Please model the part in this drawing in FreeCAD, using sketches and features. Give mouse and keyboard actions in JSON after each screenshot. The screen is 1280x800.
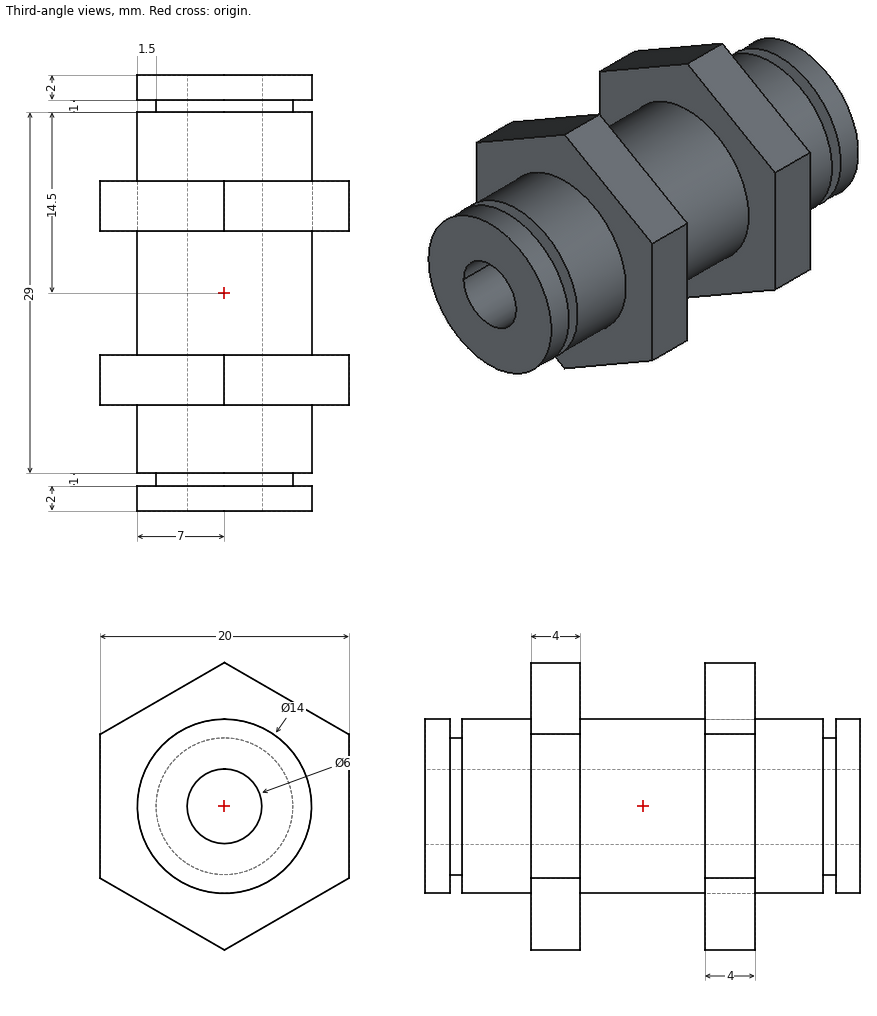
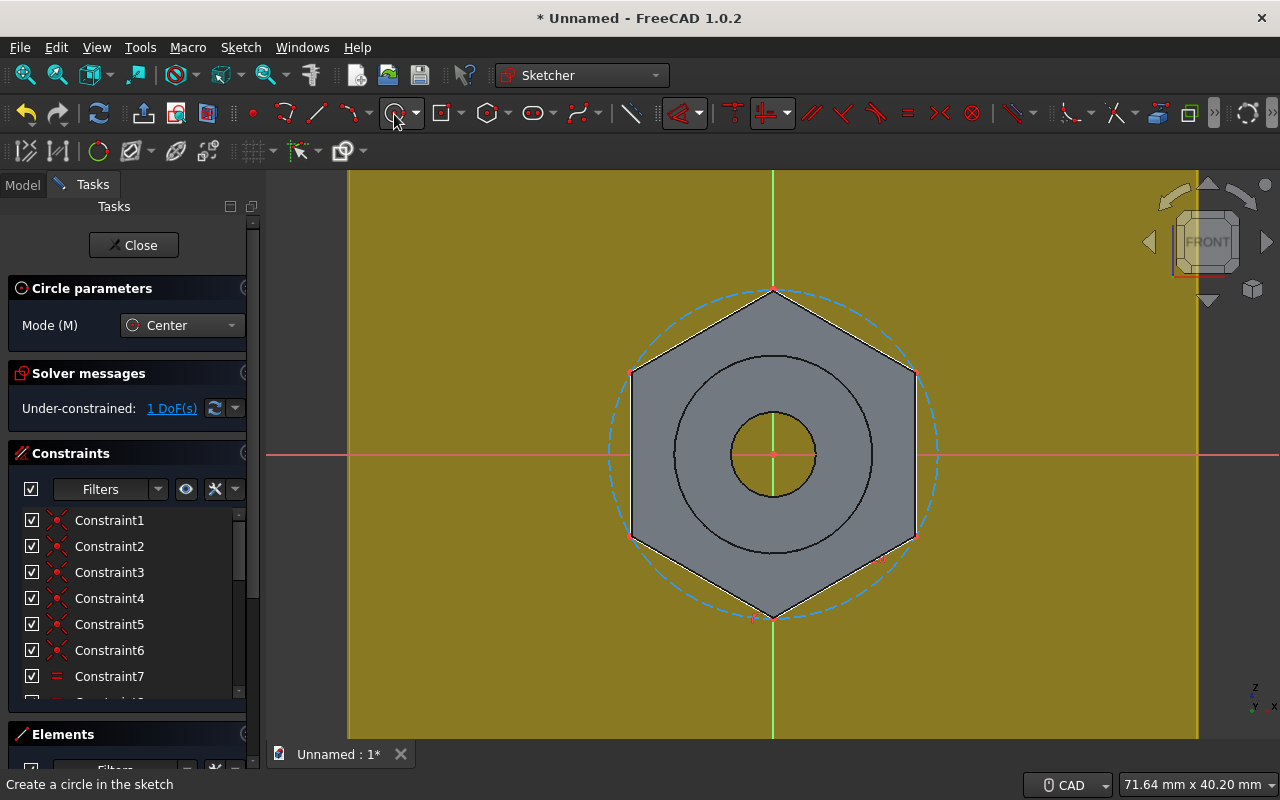
{"action": "left_click", "coordinate": [773, 455]}
{"action": "left_click", "coordinate": [843, 384]}
{"action": "key", "text": "Escape"}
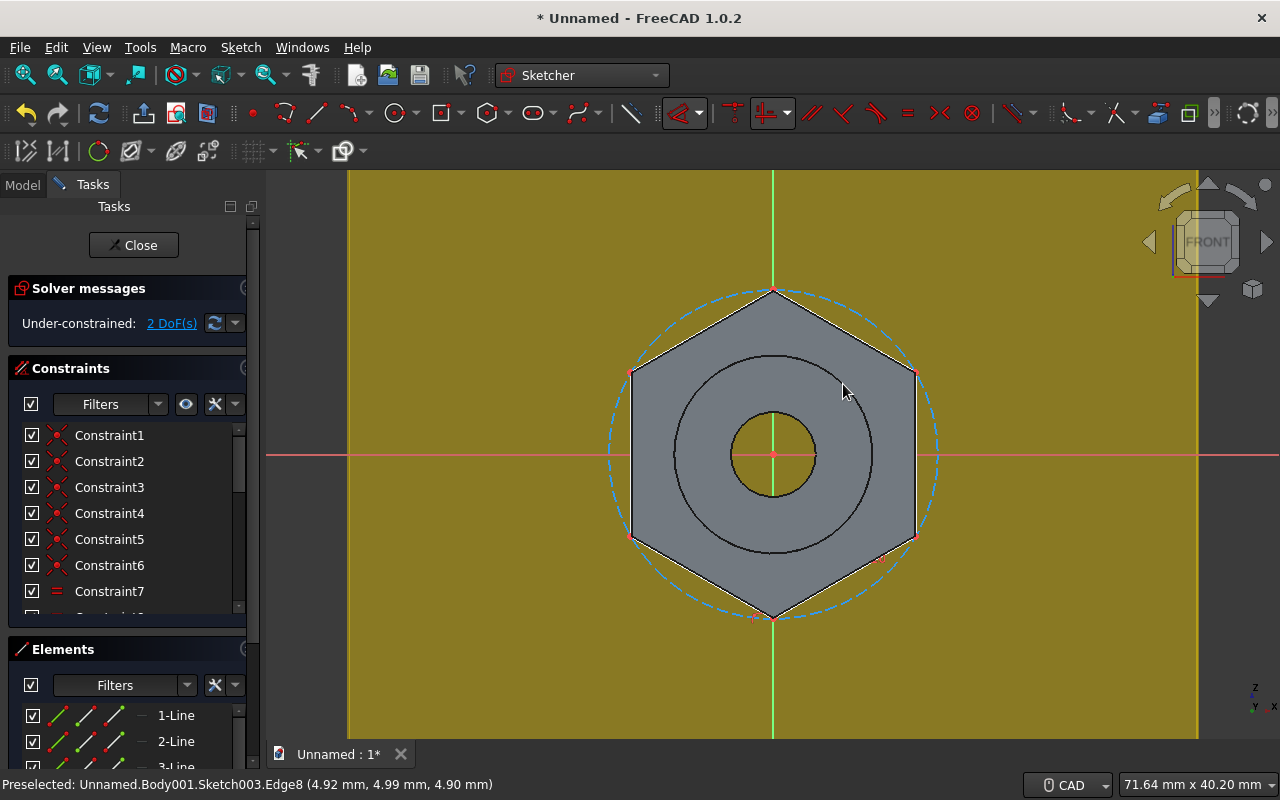
{"action": "left_click", "coordinate": [843, 385]}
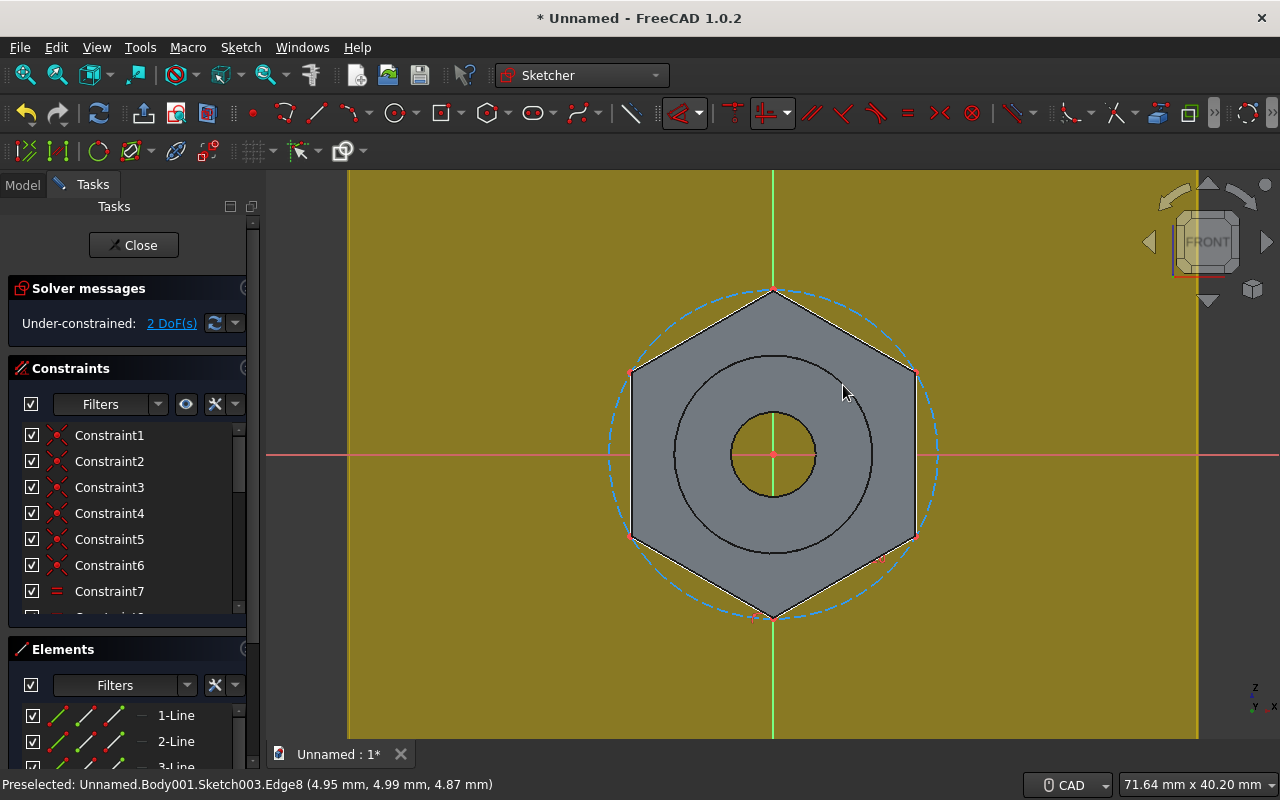
{"action": "key", "text": "k o"}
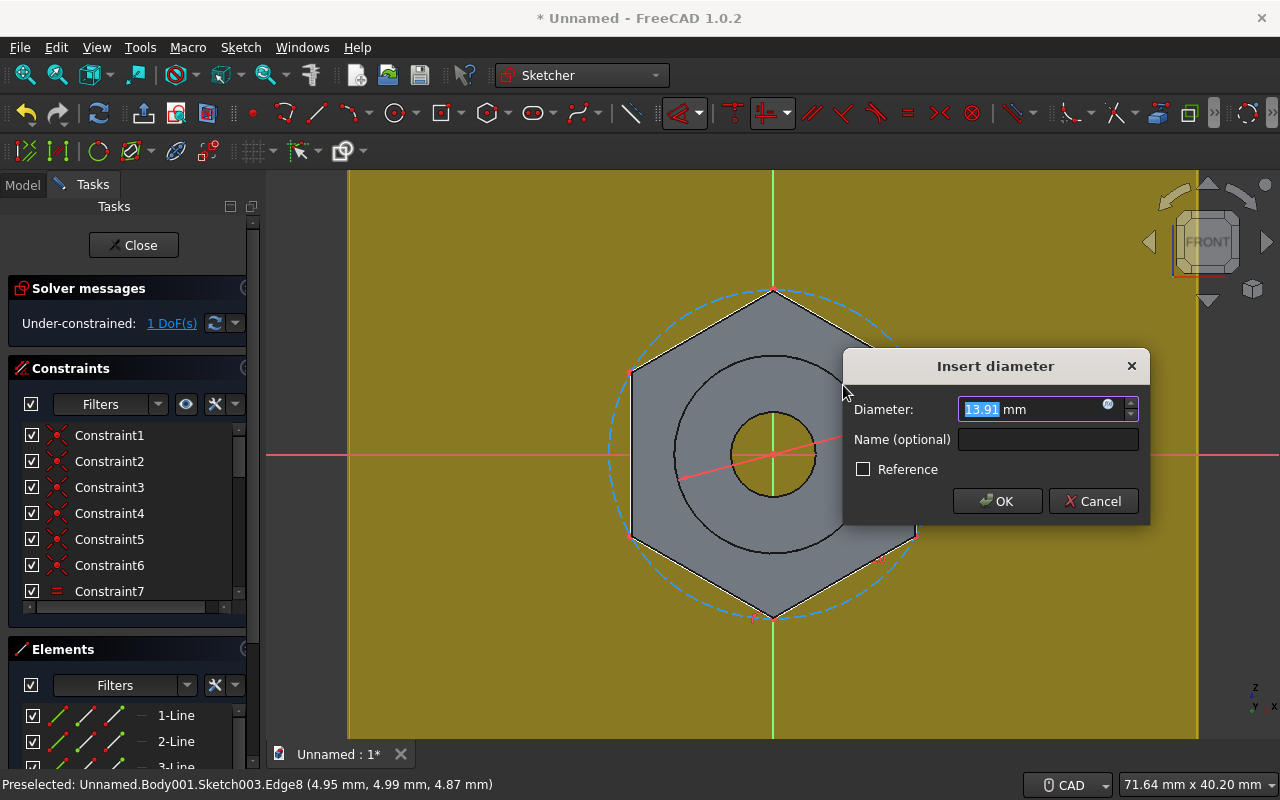
{"action": "type", "text": "14"}
{"action": "key", "text": "Return"}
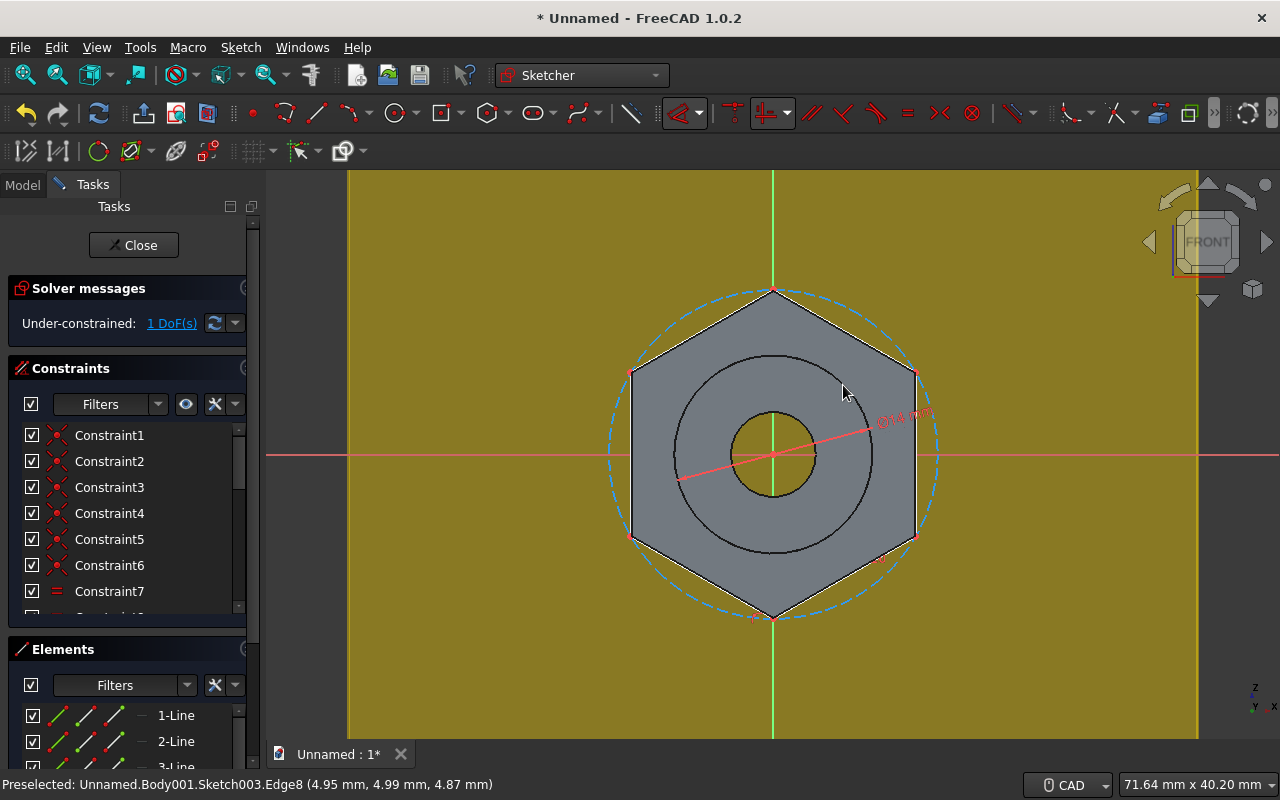
{"action": "left_click", "coordinate": [631, 372]}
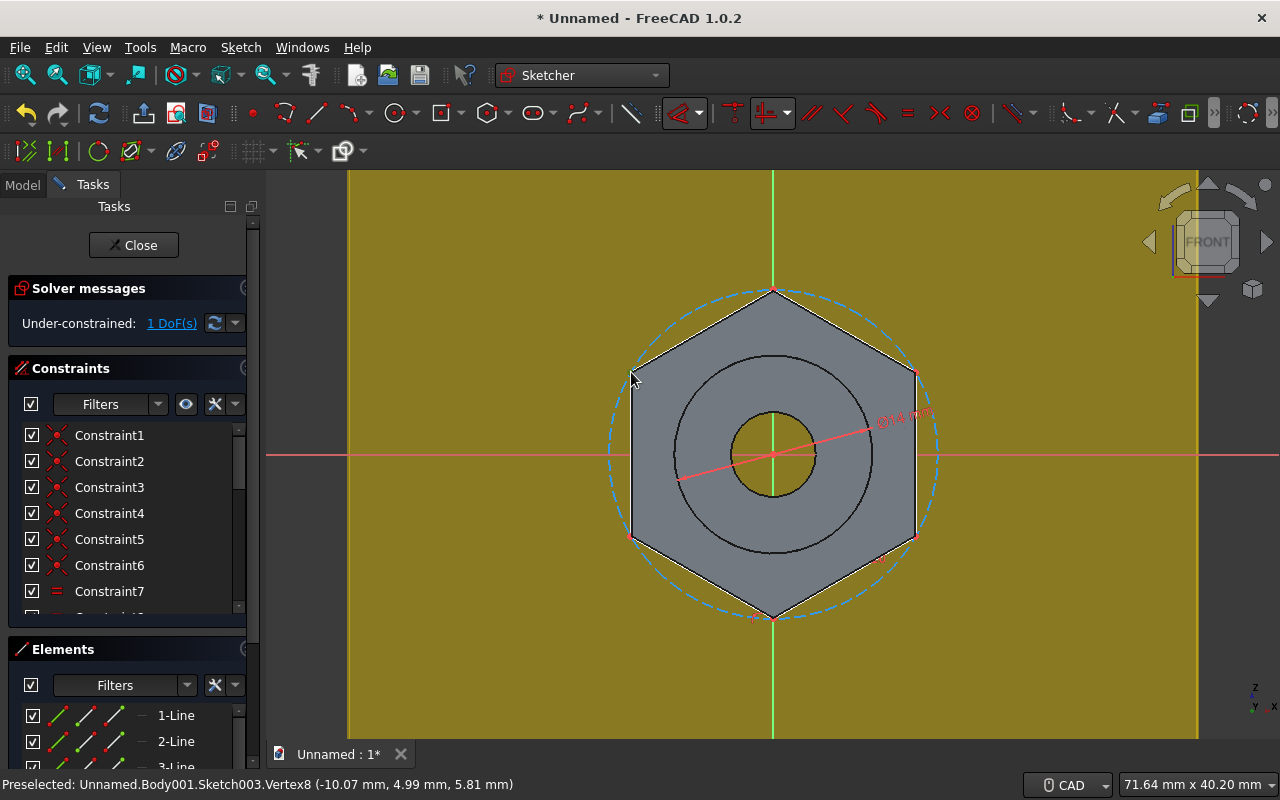
{"action": "left_click", "coordinate": [916, 537]}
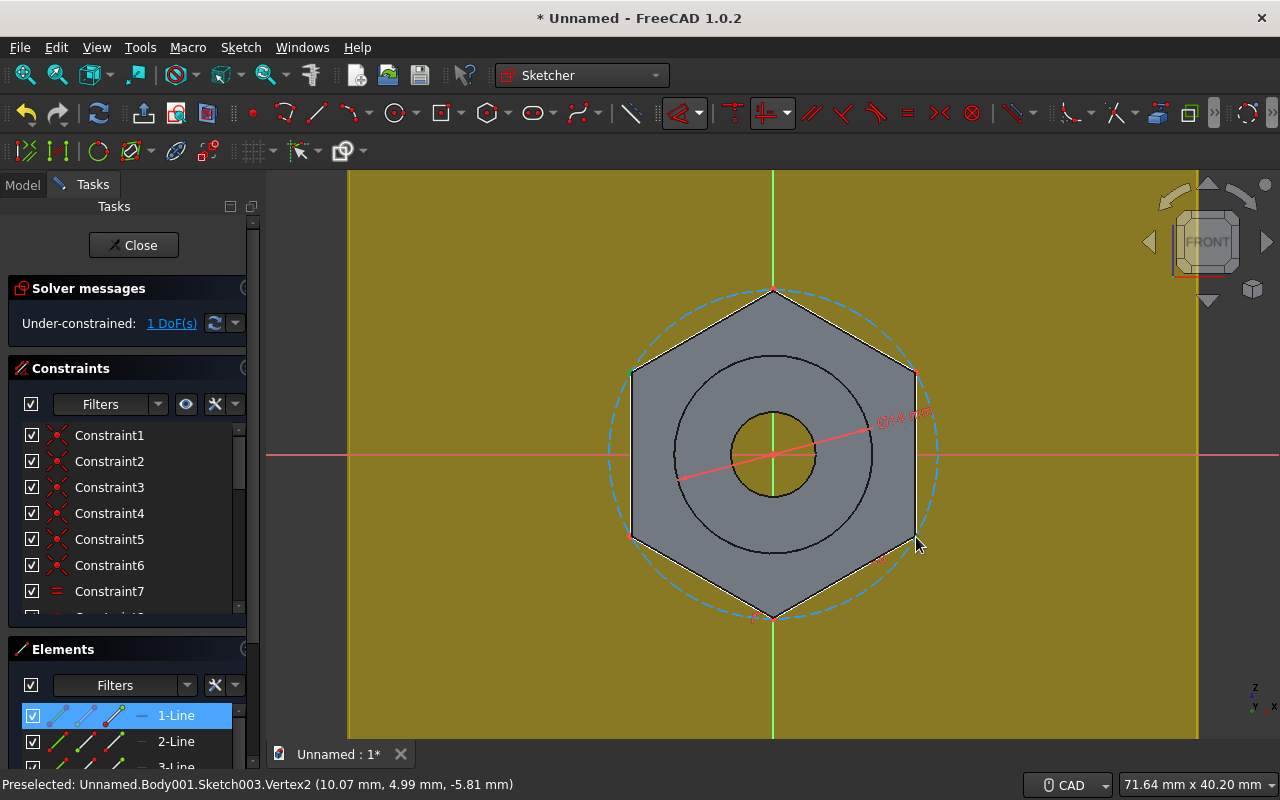
{"action": "left_click", "coordinate": [702, 114]}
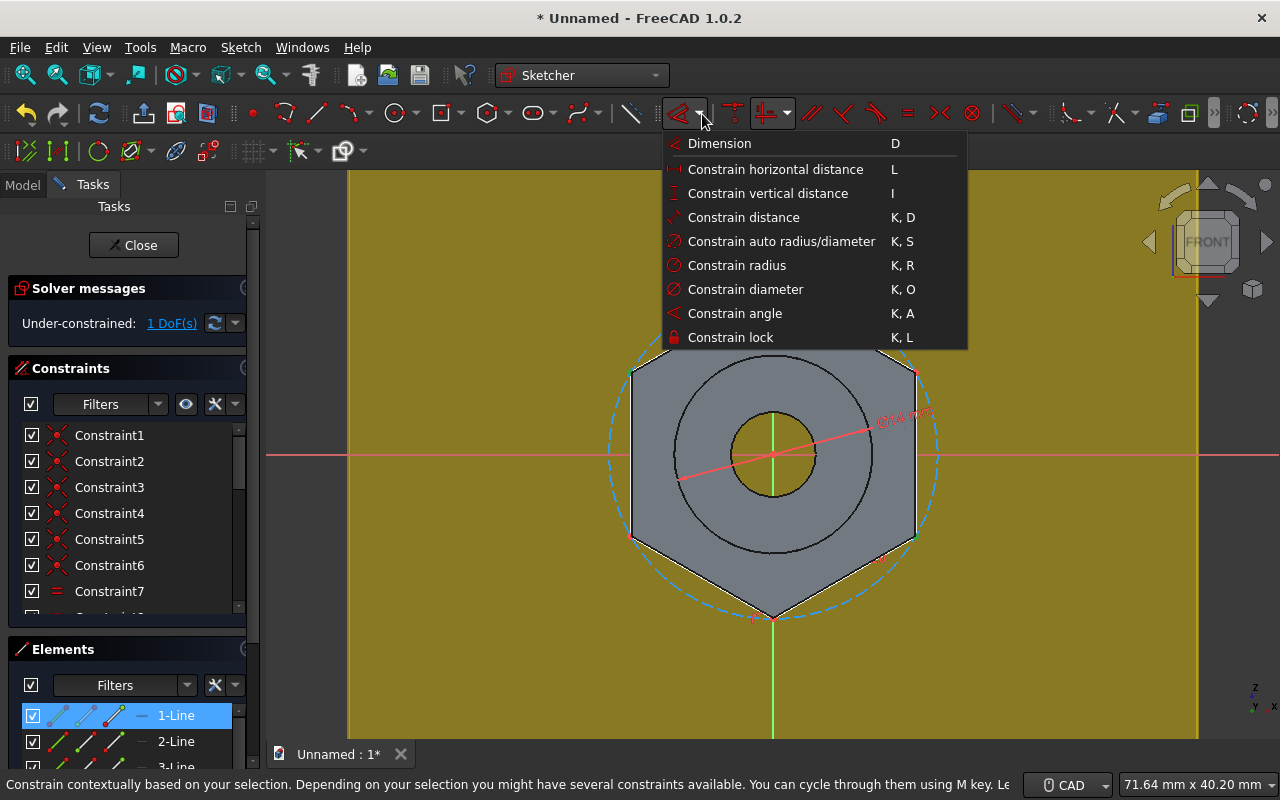
{"action": "left_click", "coordinate": [815, 169]}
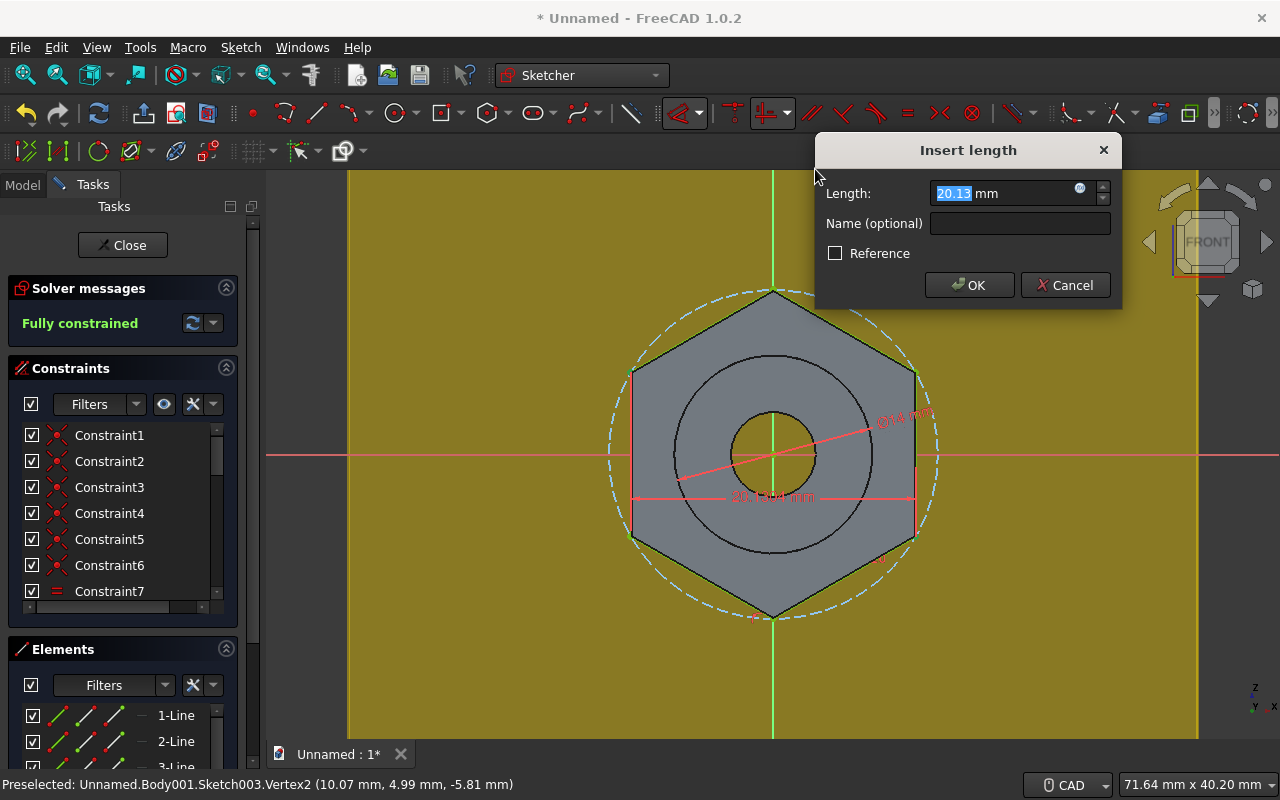
{"action": "type", "text": "20"}
{"action": "key", "text": "Return"}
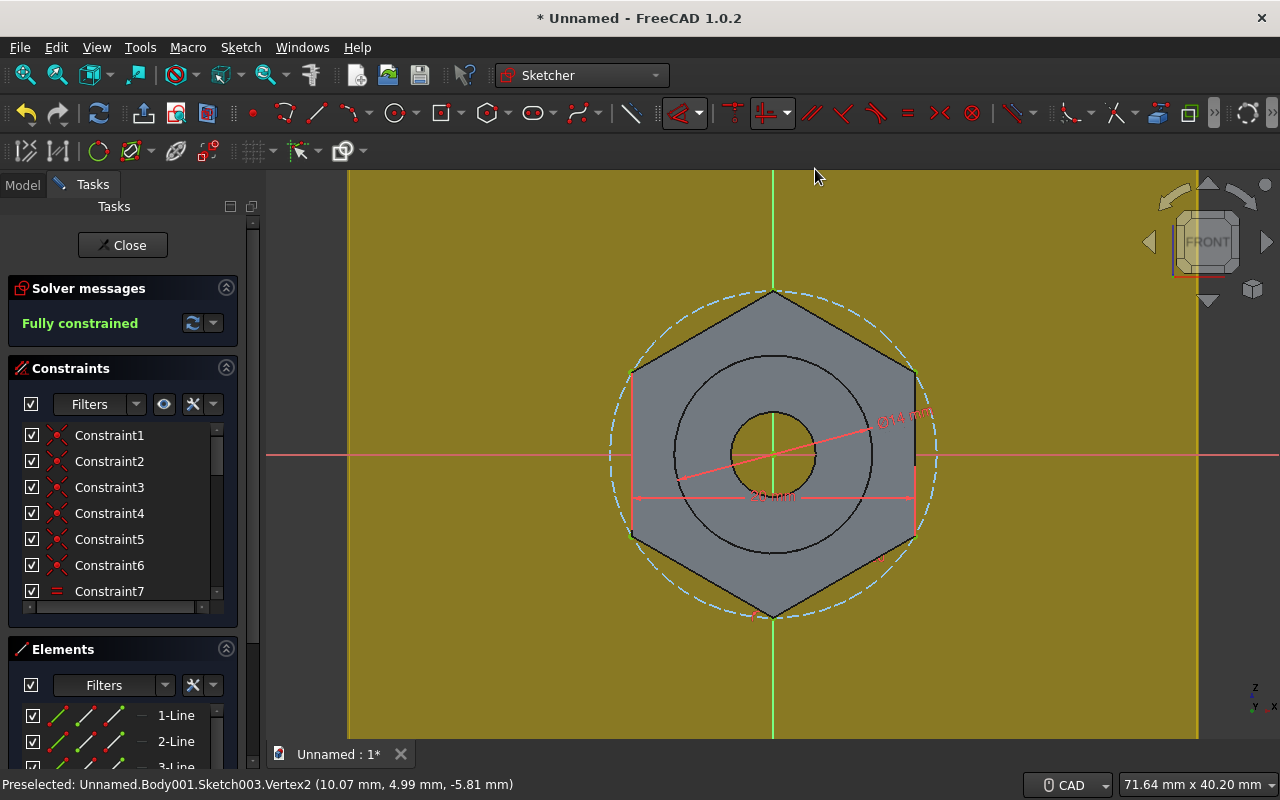
{"action": "left_click", "coordinate": [123, 245]}